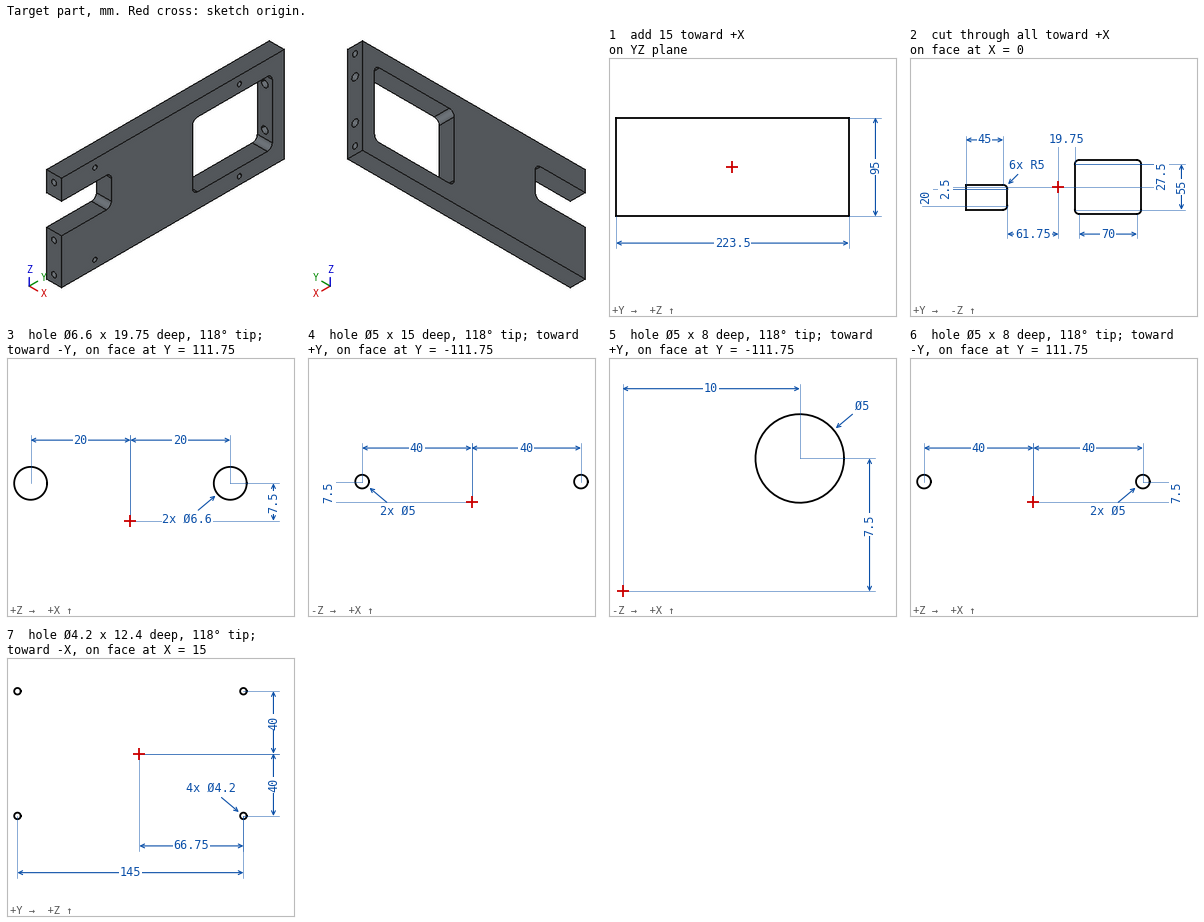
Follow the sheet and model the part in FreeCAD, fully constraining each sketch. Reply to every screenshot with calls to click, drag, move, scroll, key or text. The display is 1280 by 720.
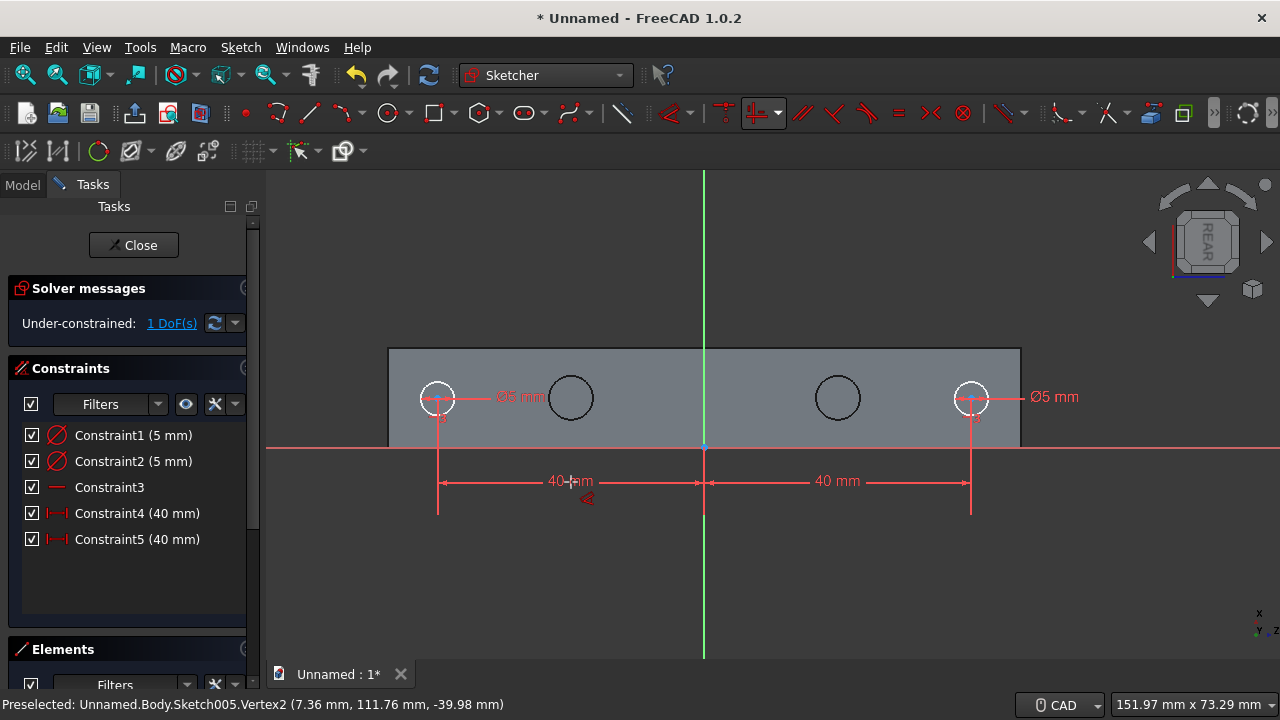
click(971, 399)
click(1005, 423)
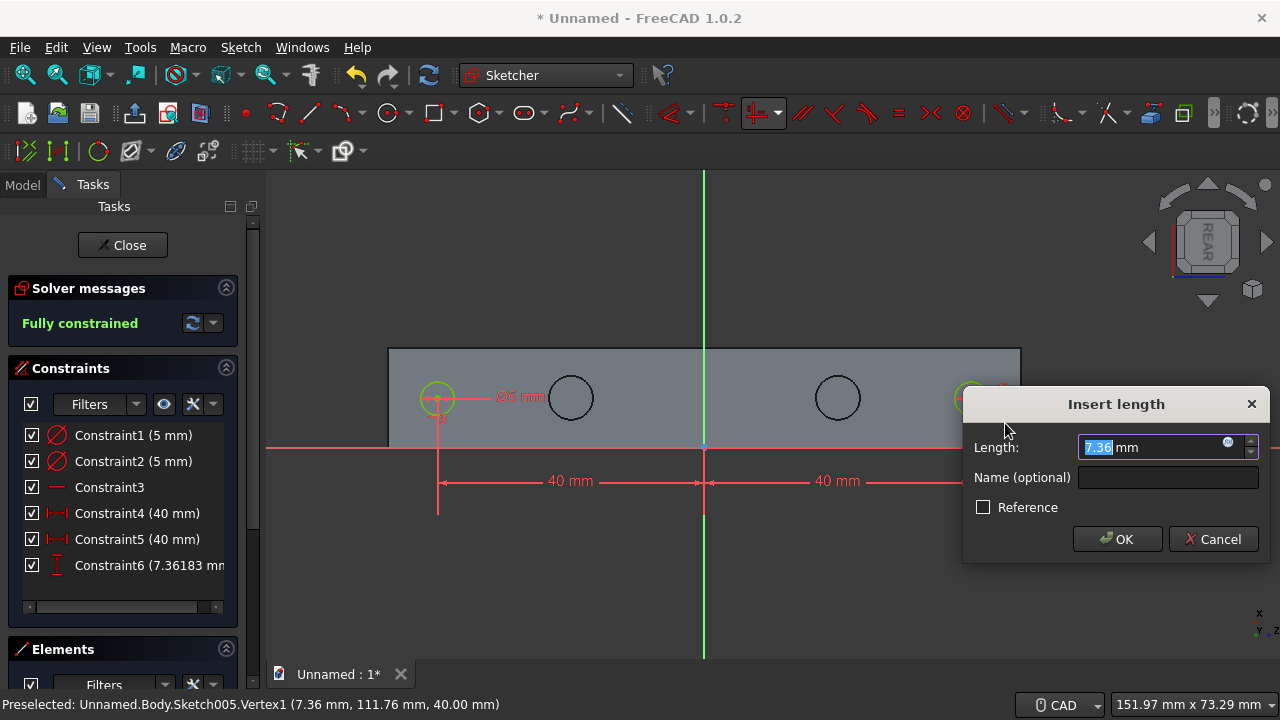
text(7.5)
key(Return)
key(Escape)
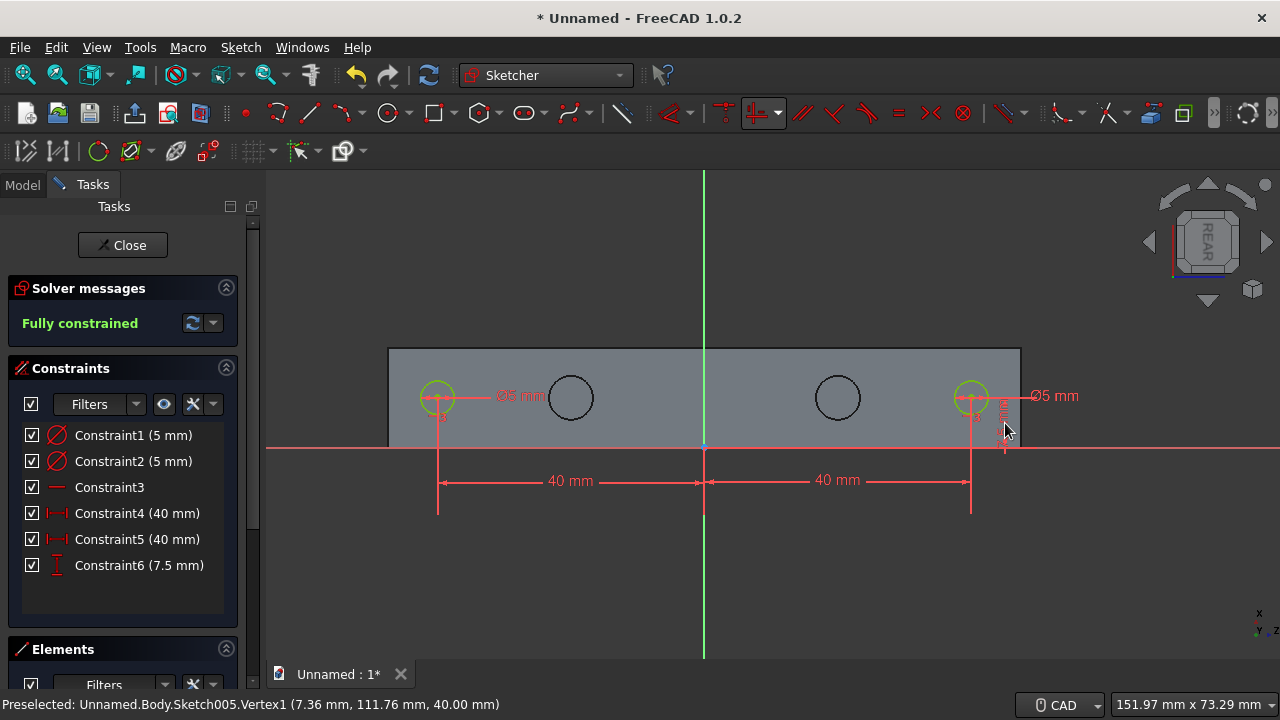
click(123, 245)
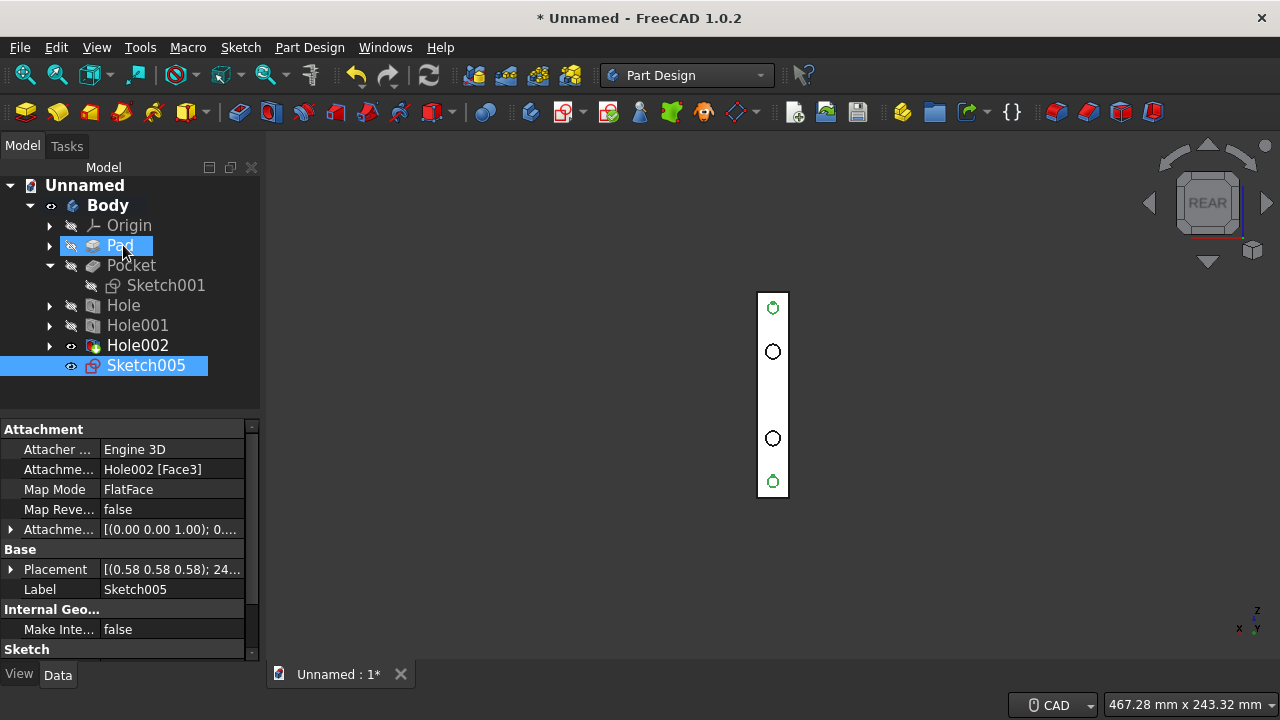
click(272, 112)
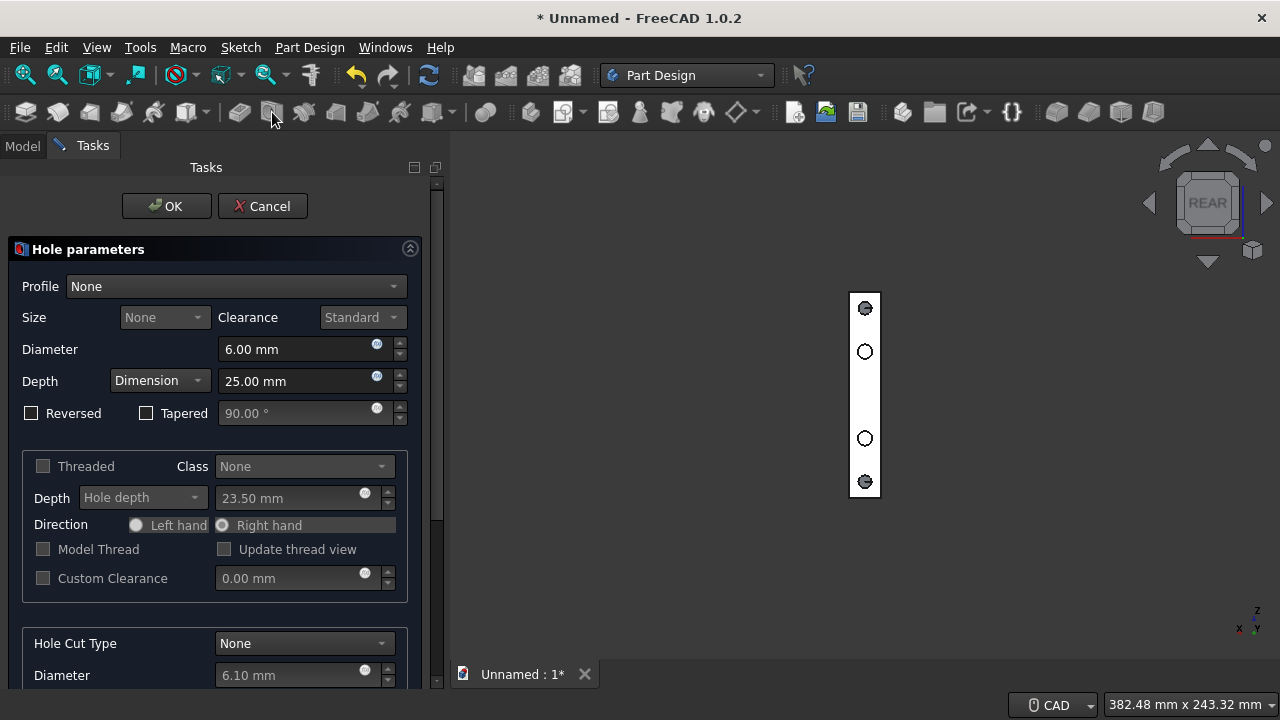
triple_click(305, 349)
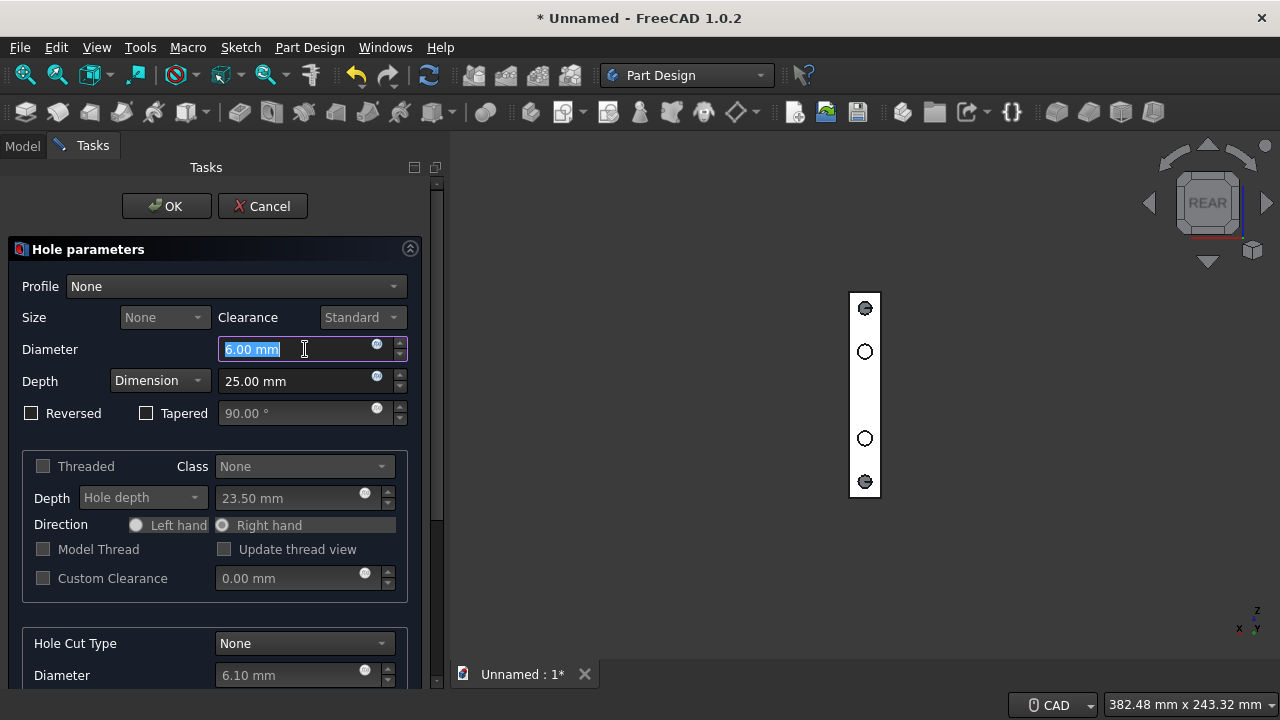
text(5)
key(Tab)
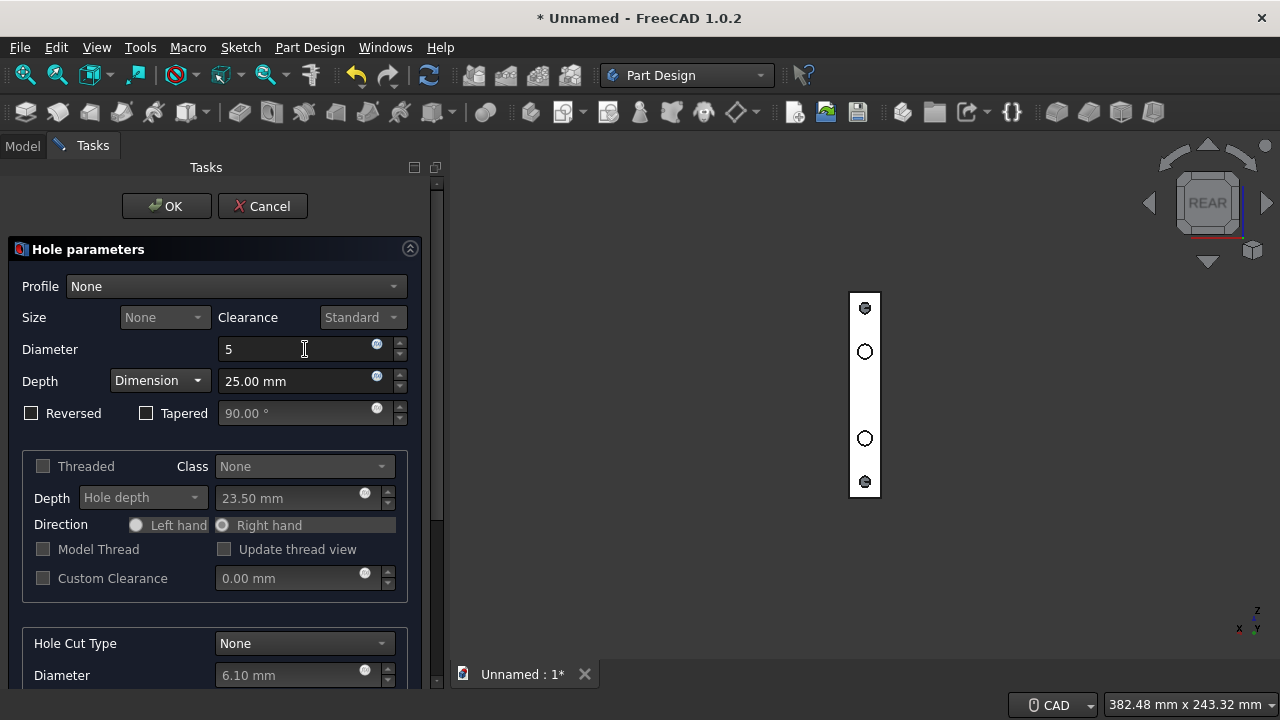
triple_click(305, 381)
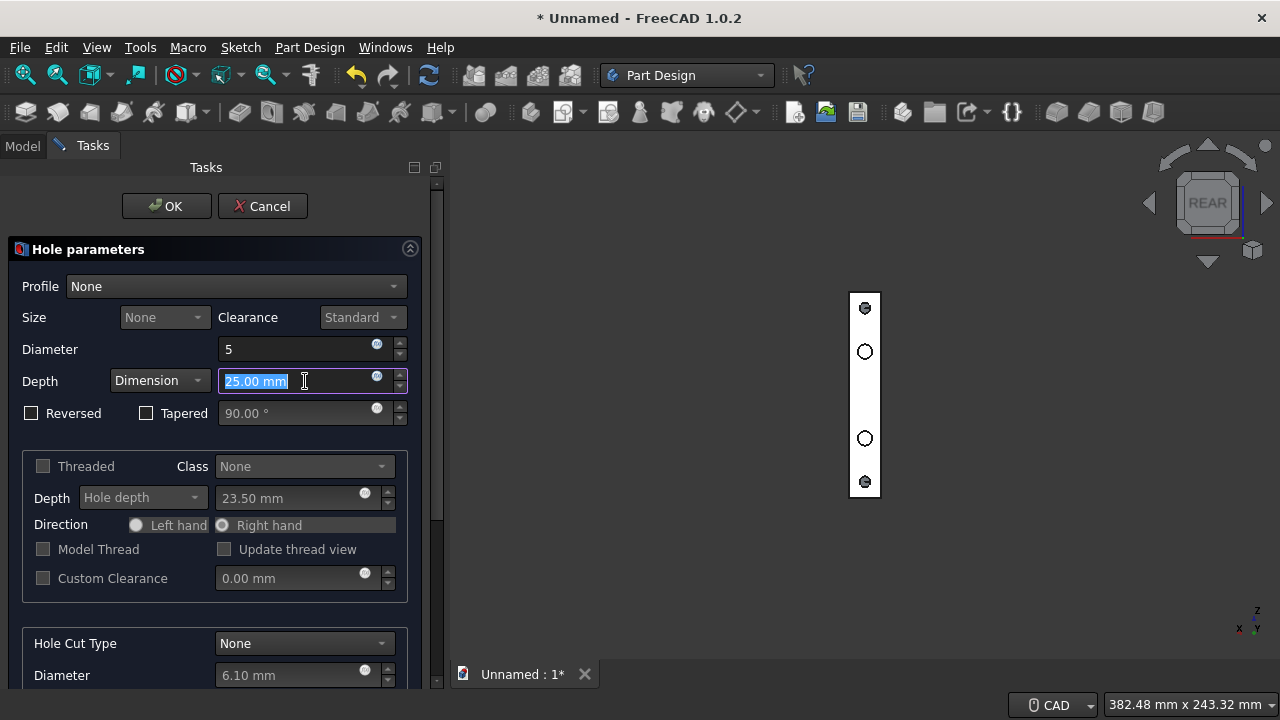
text(8)
key(Tab)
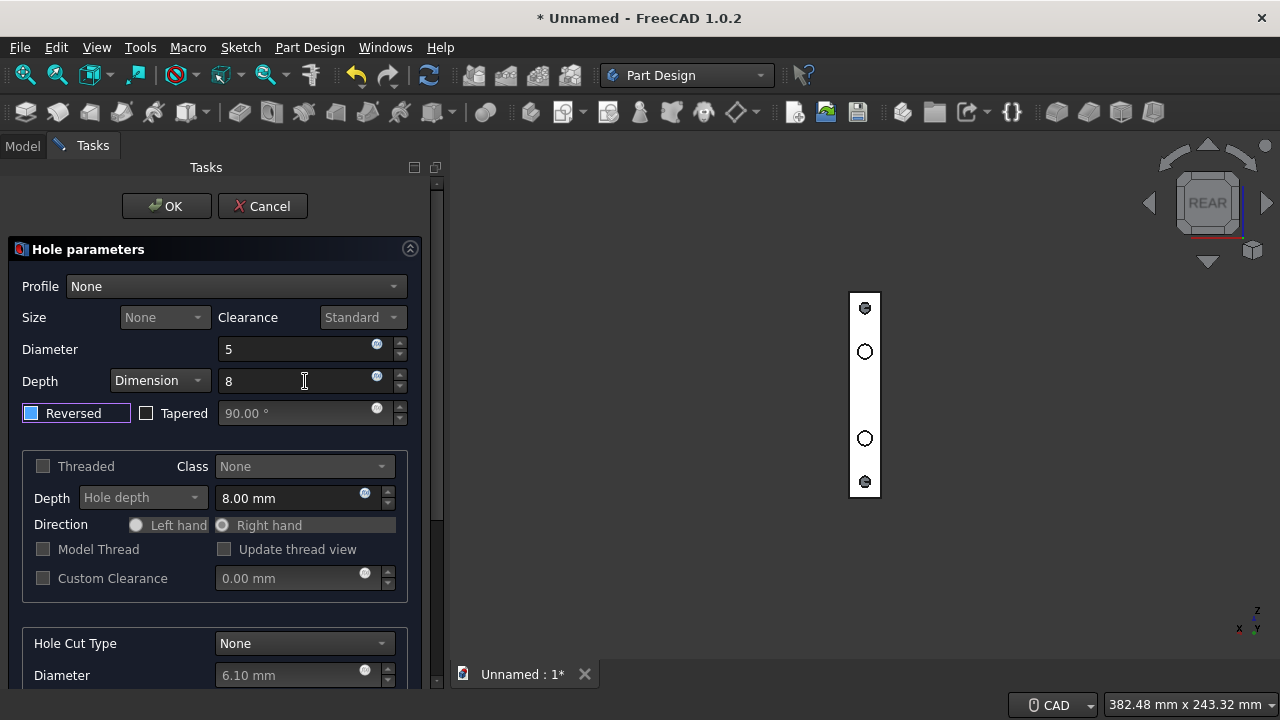
click(167, 206)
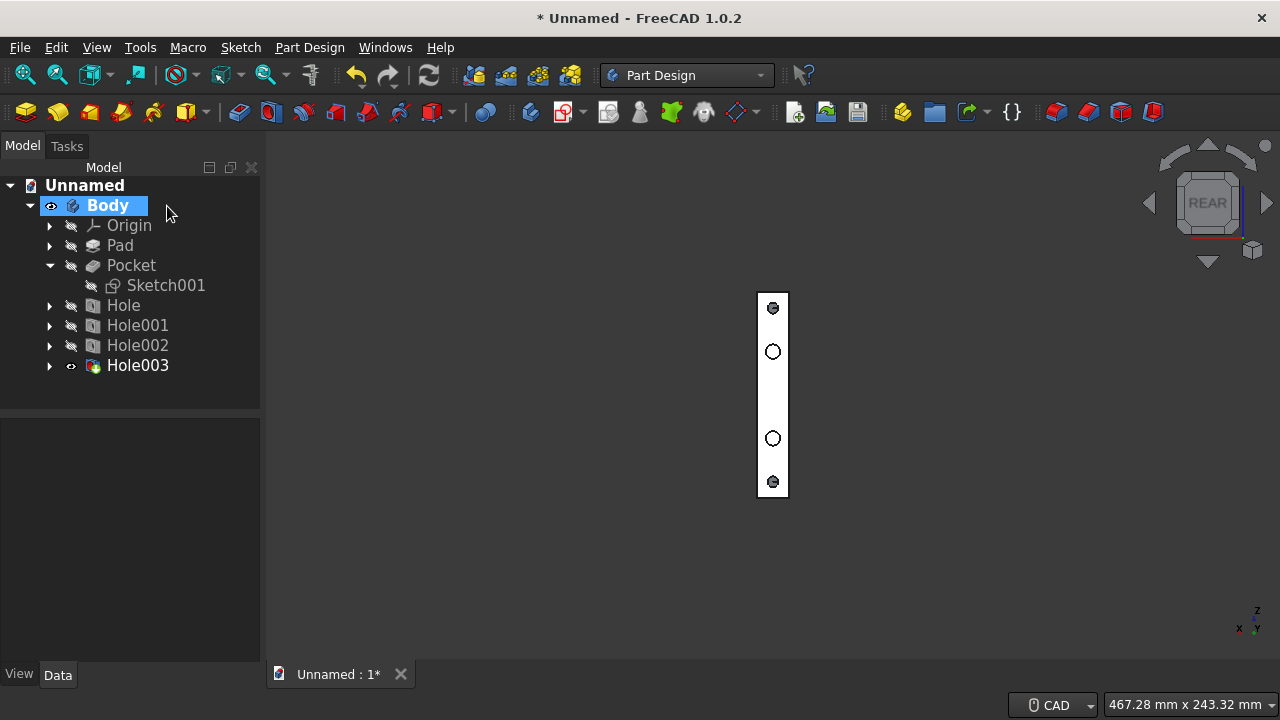
click(26, 76)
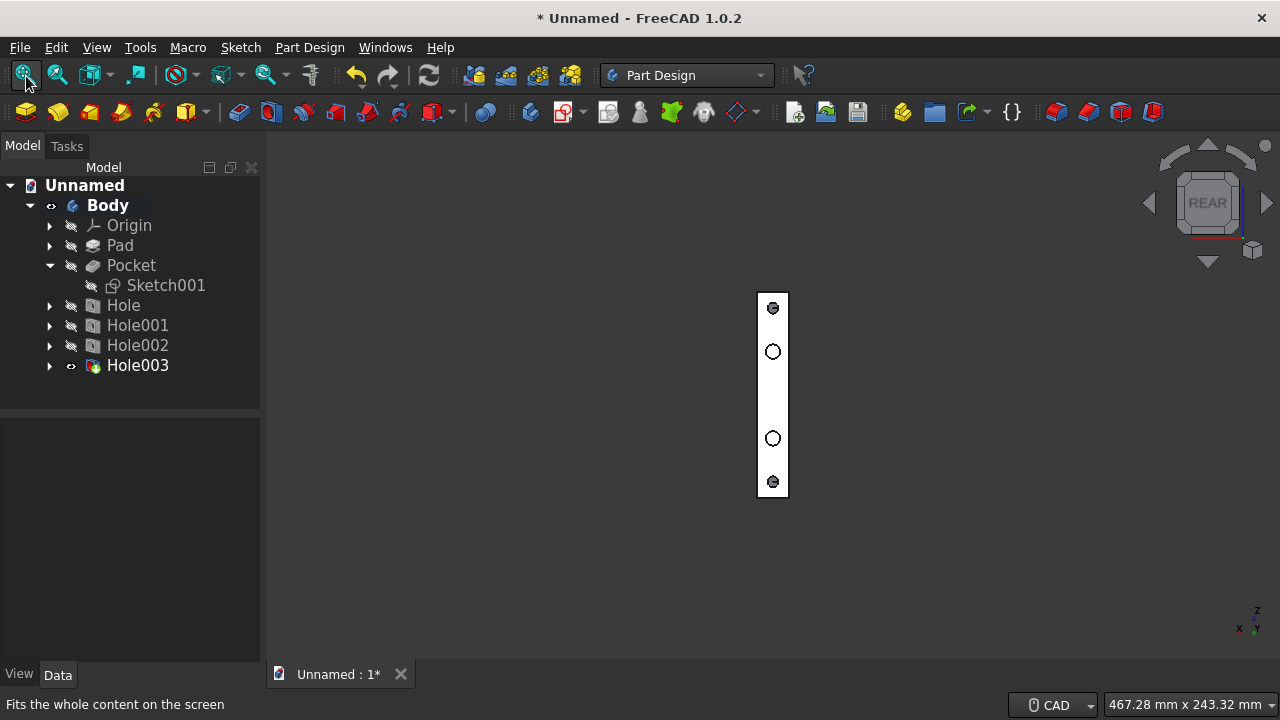
key(0)